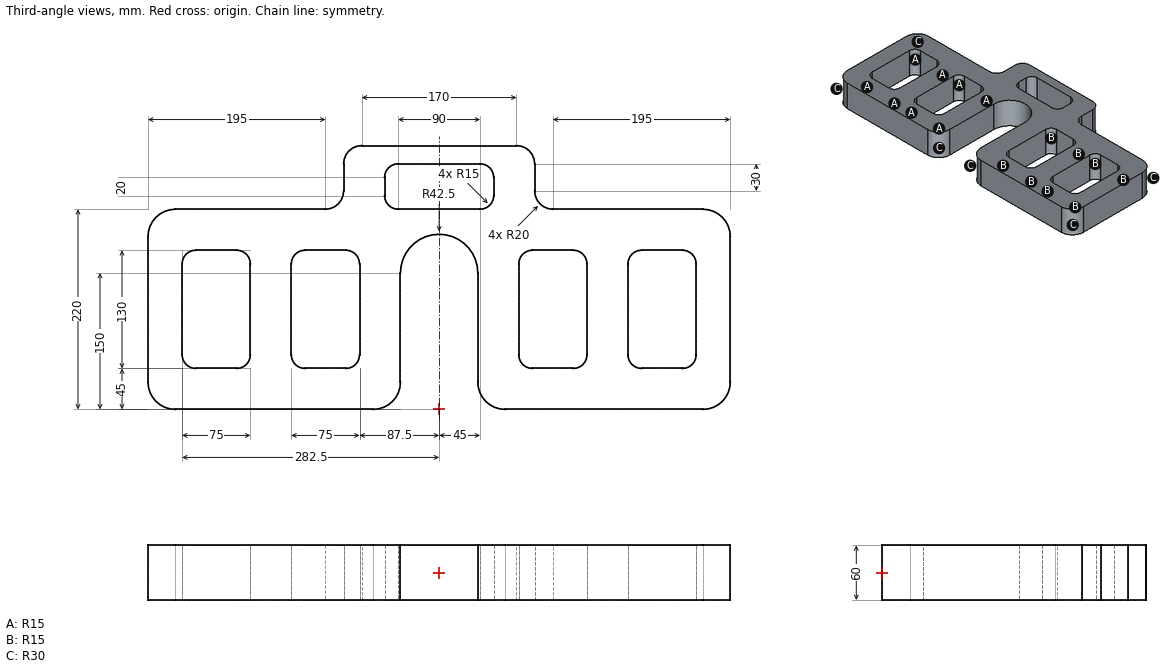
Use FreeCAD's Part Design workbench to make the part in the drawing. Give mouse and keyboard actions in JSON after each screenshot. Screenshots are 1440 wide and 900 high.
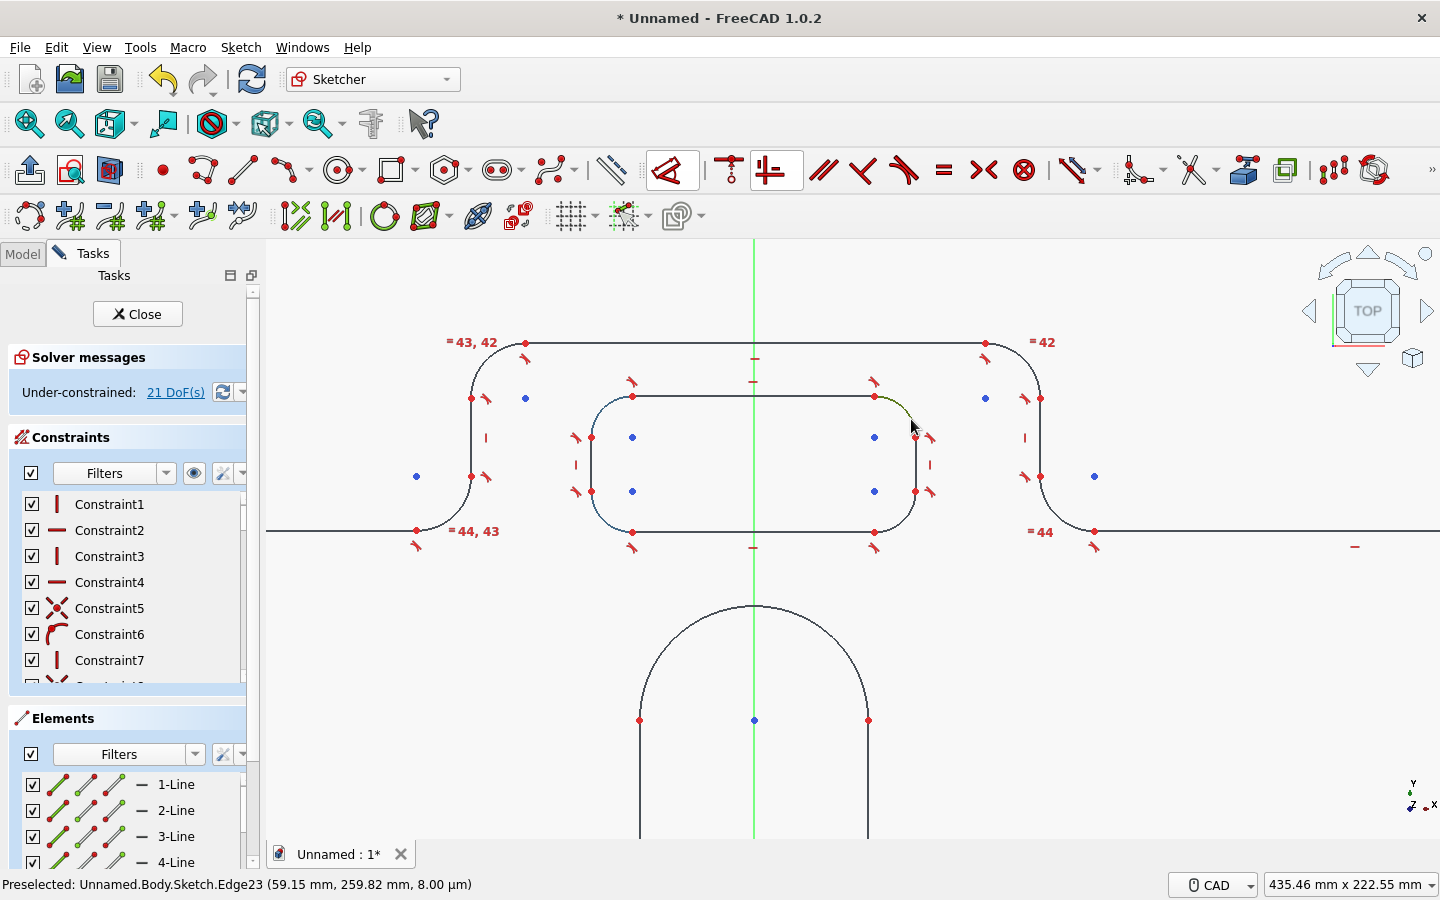
{"action": "left_click", "coordinate": [893, 528]}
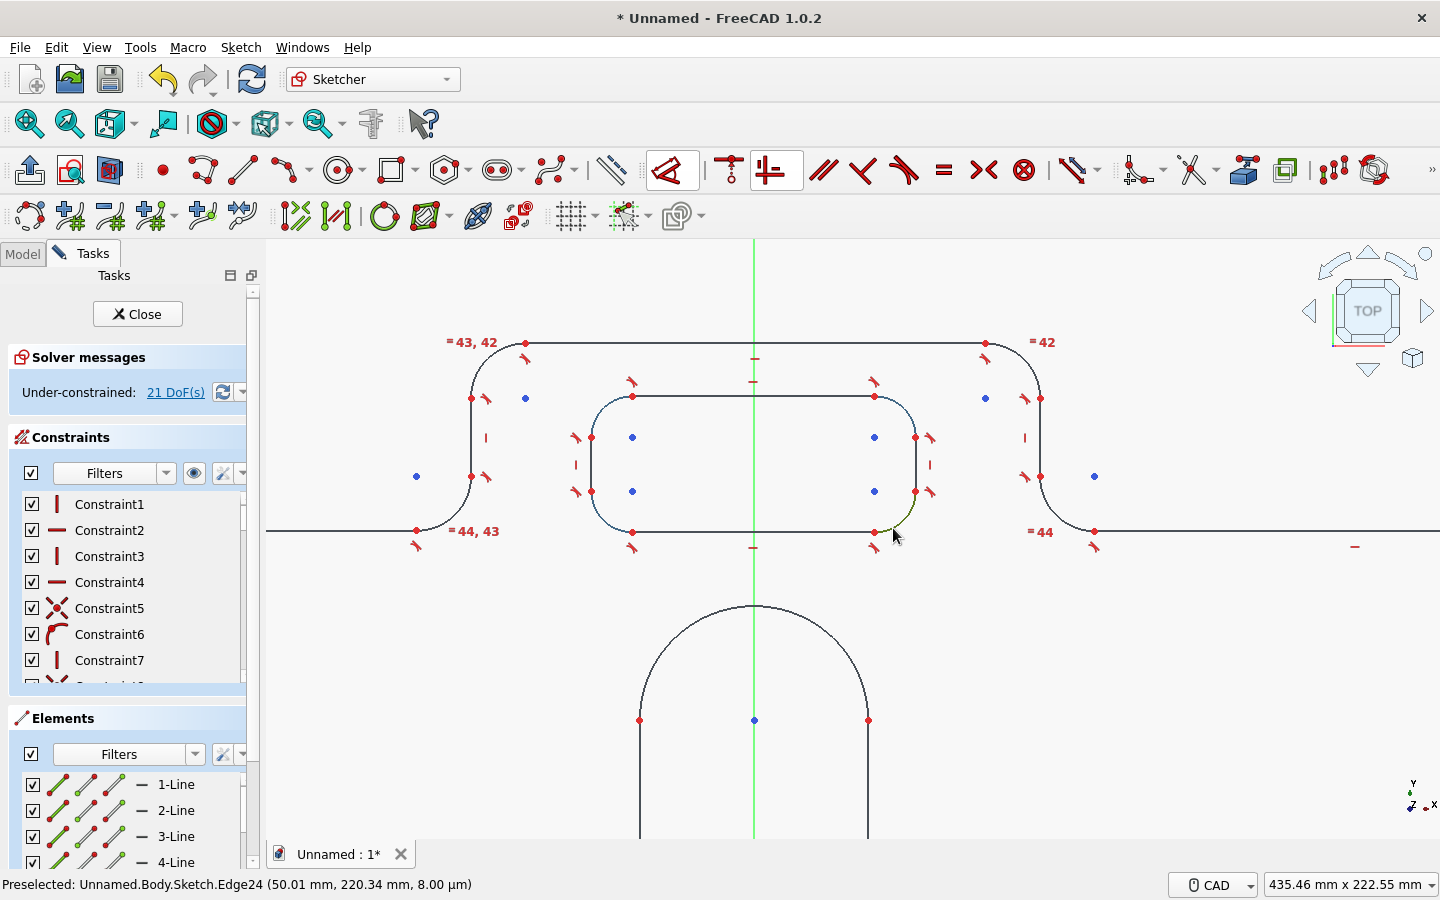
{"action": "key", "text": "e"}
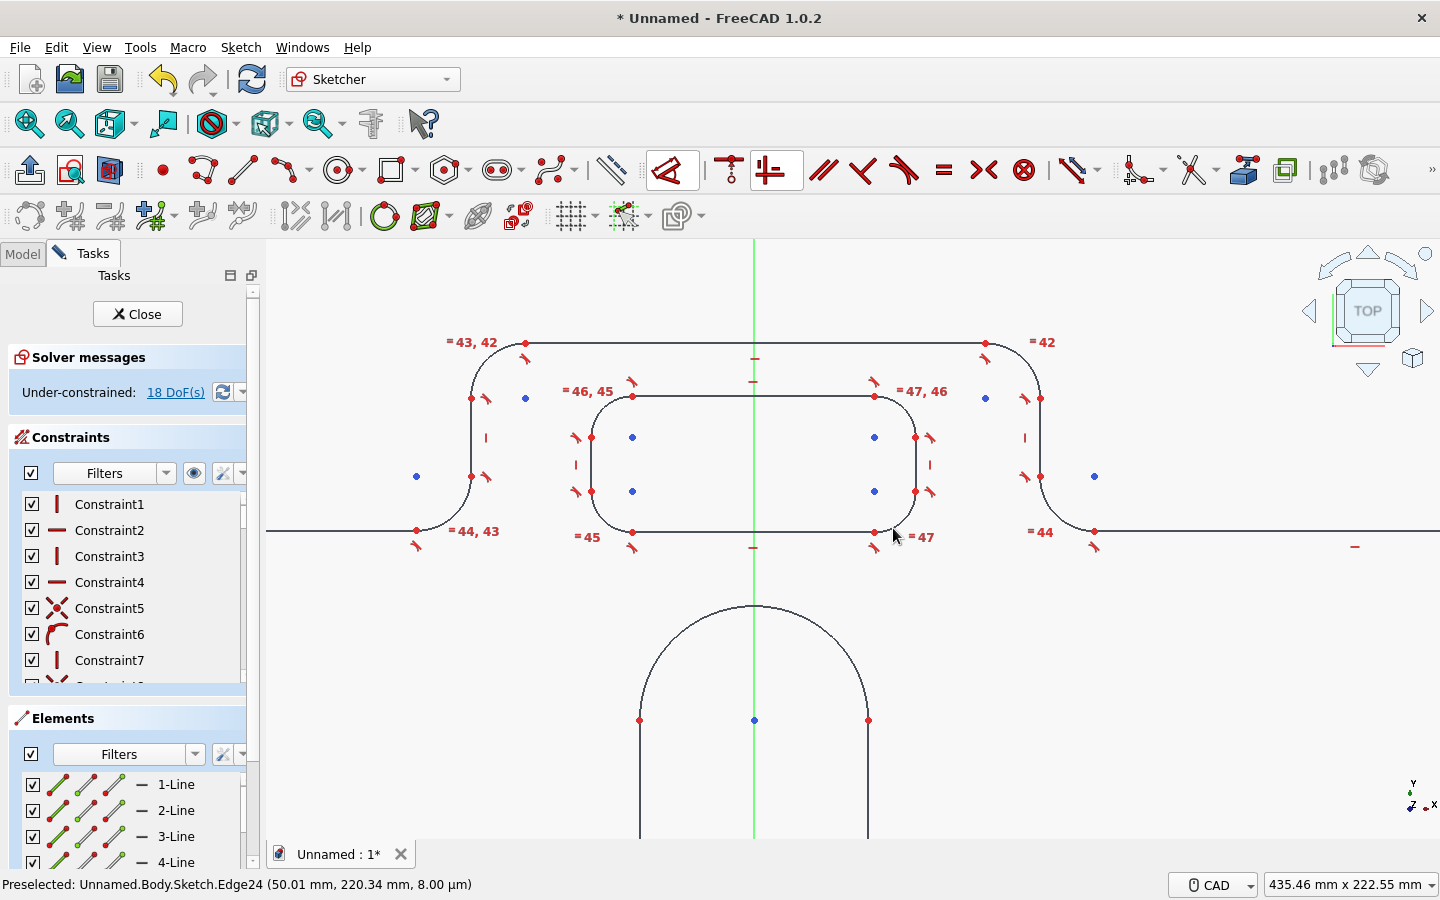
{"action": "left_click", "coordinate": [754, 720]}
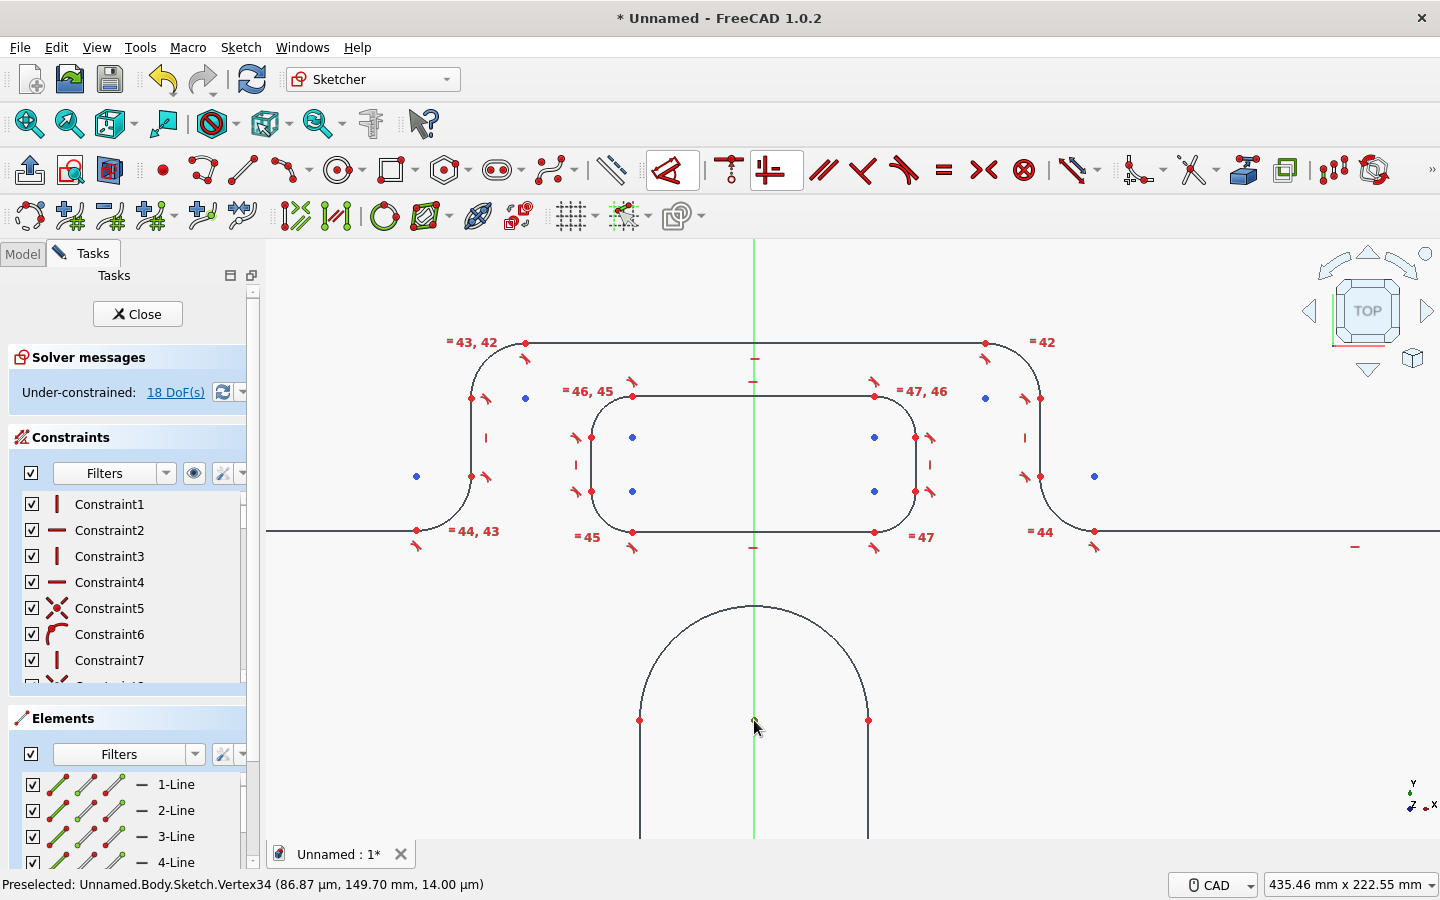
{"action": "left_click", "coordinate": [754, 772]}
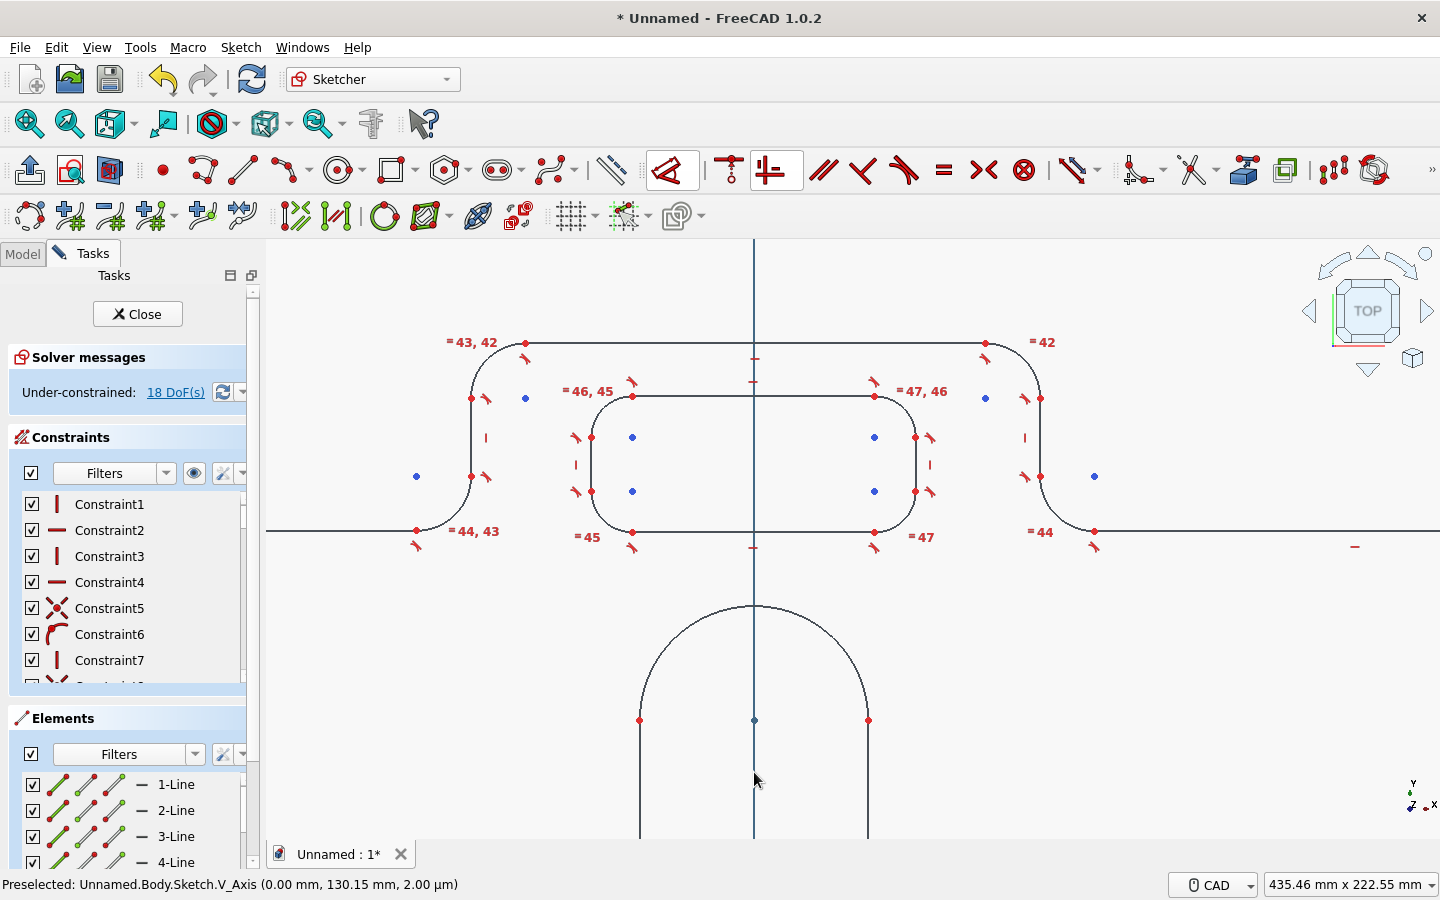
{"action": "left_click", "coordinate": [730, 170]}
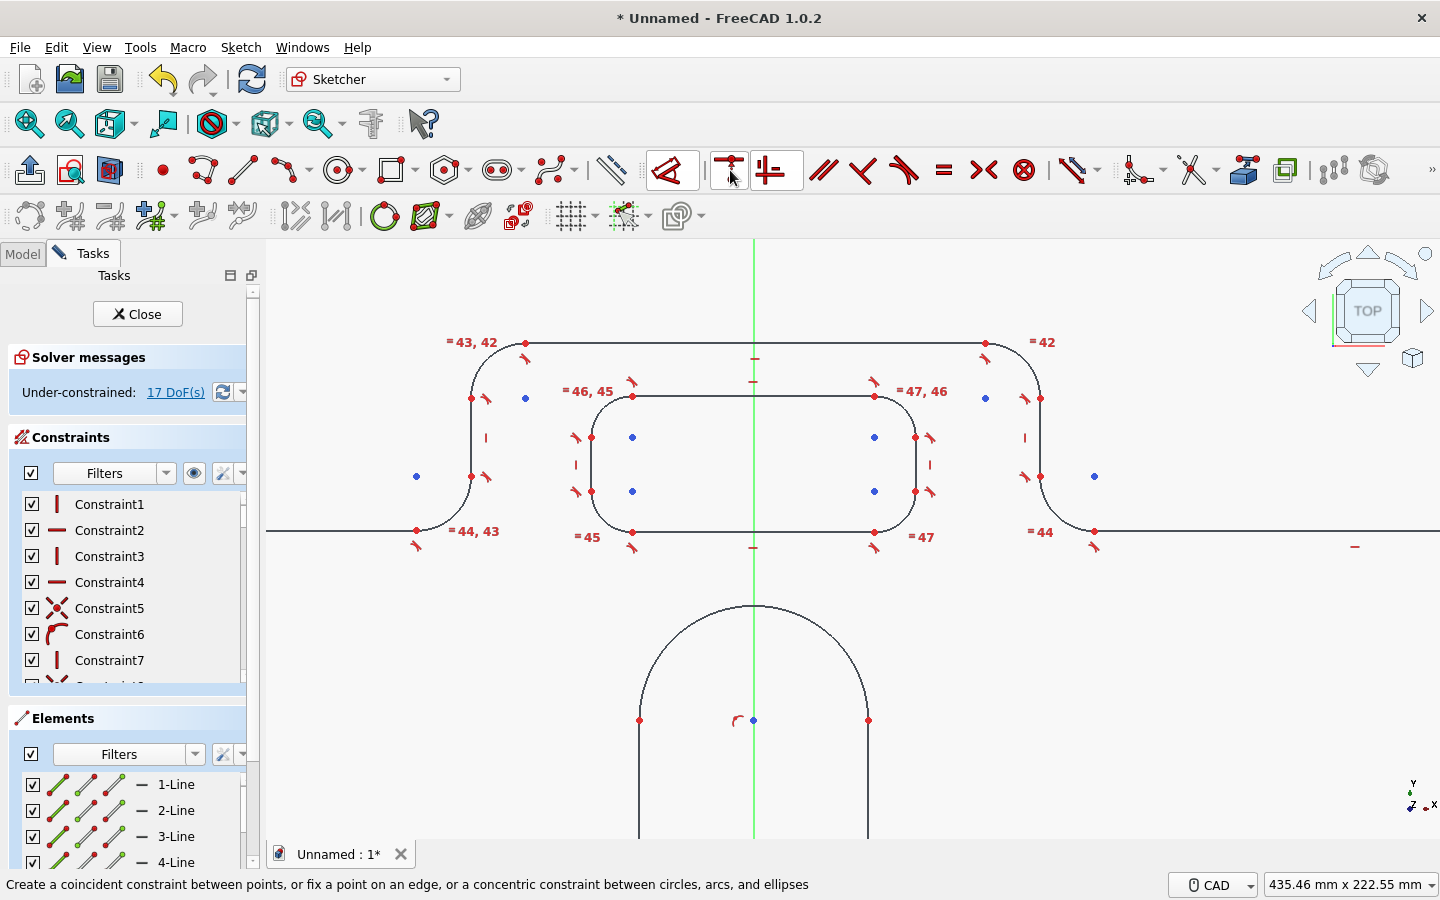
{"action": "left_click", "coordinate": [416, 476]}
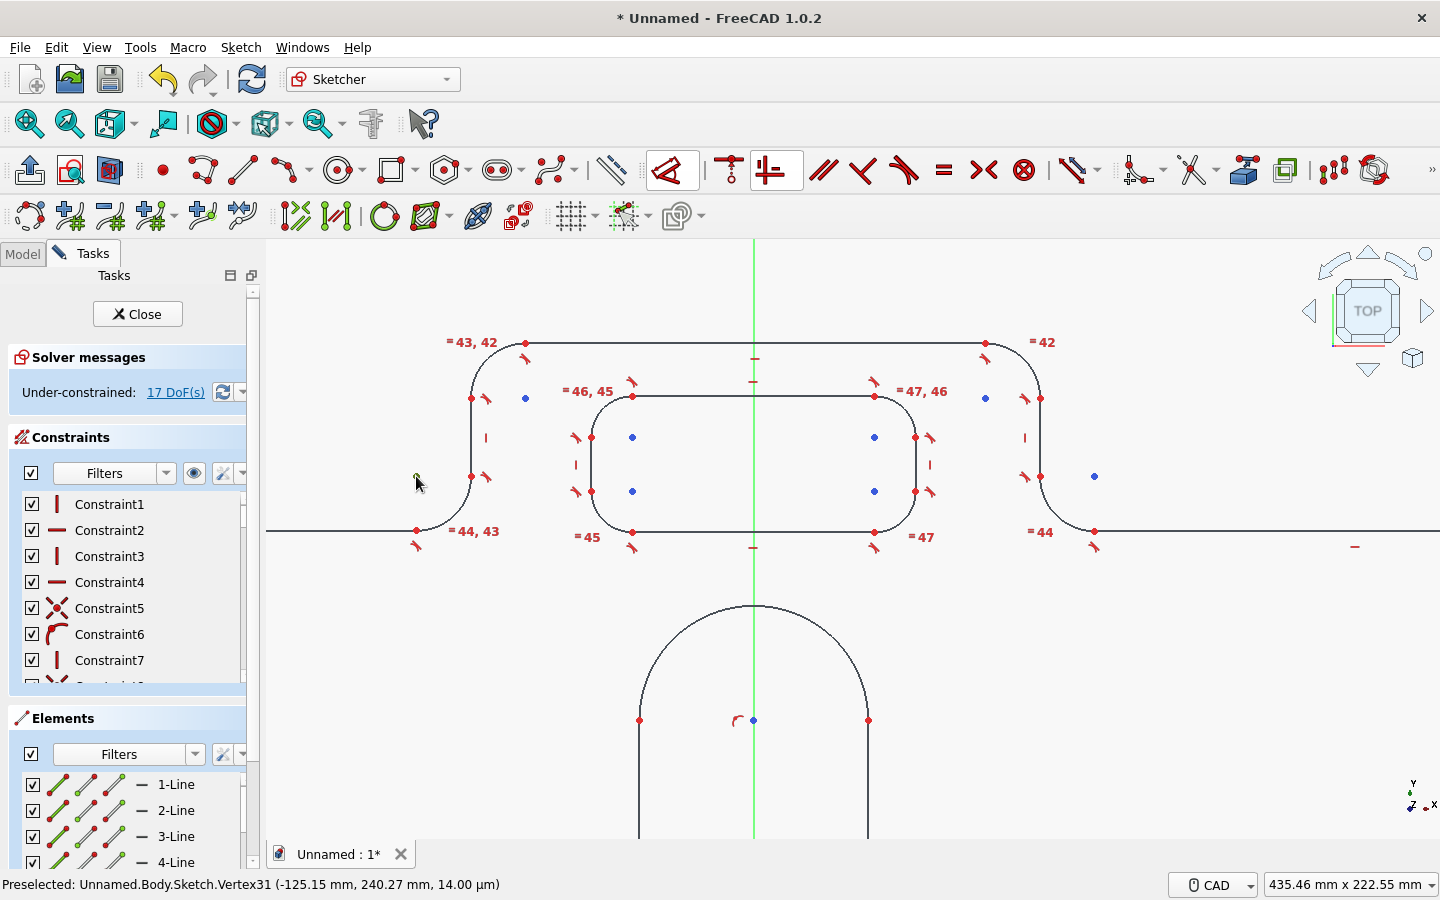
{"action": "left_click", "coordinate": [1095, 476]}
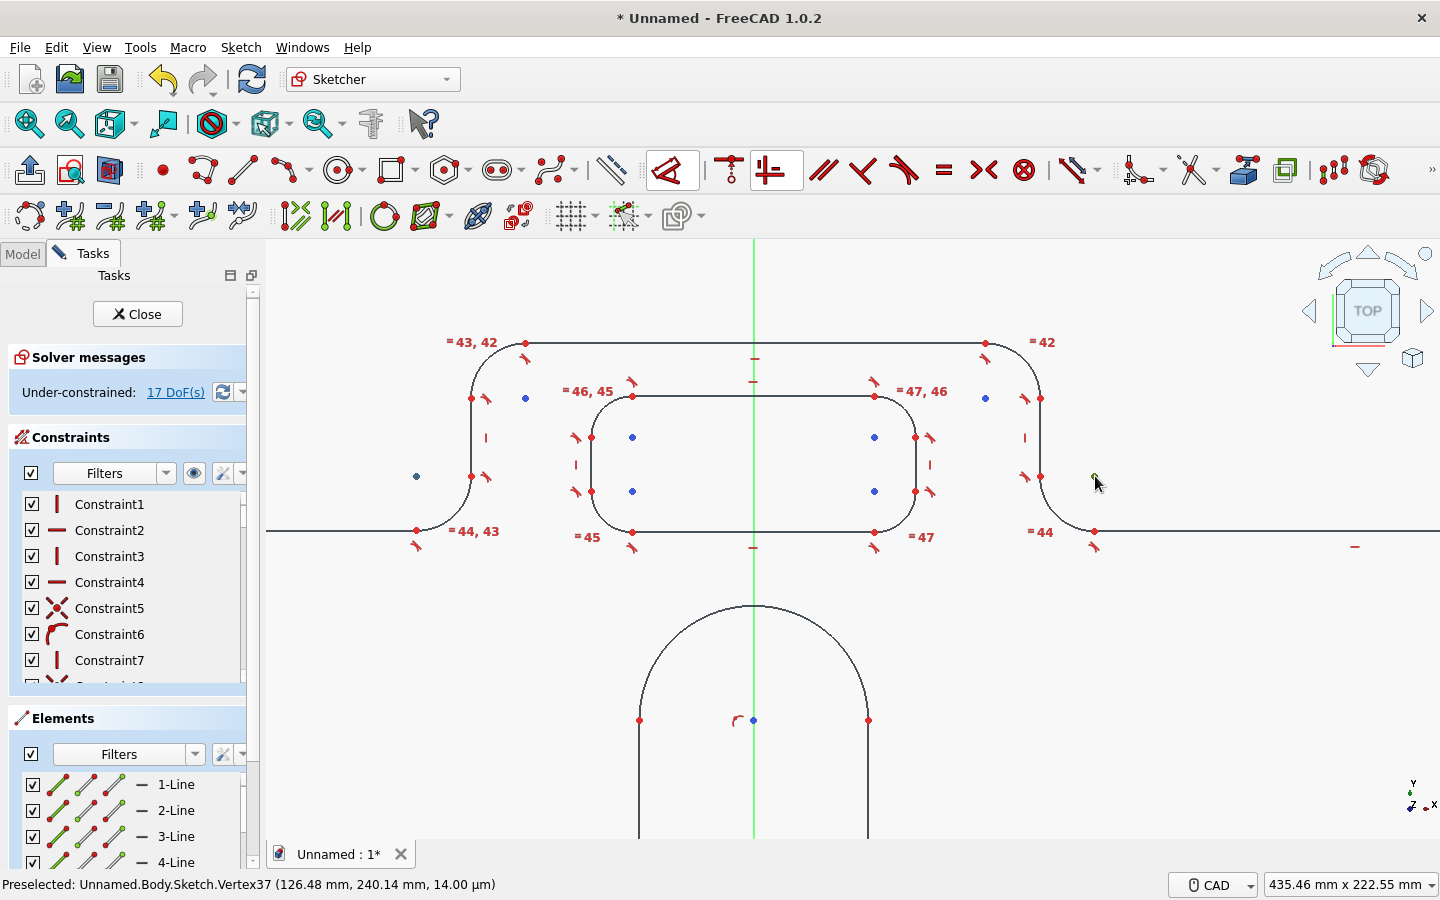
{"action": "left_click", "coordinate": [754, 772]}